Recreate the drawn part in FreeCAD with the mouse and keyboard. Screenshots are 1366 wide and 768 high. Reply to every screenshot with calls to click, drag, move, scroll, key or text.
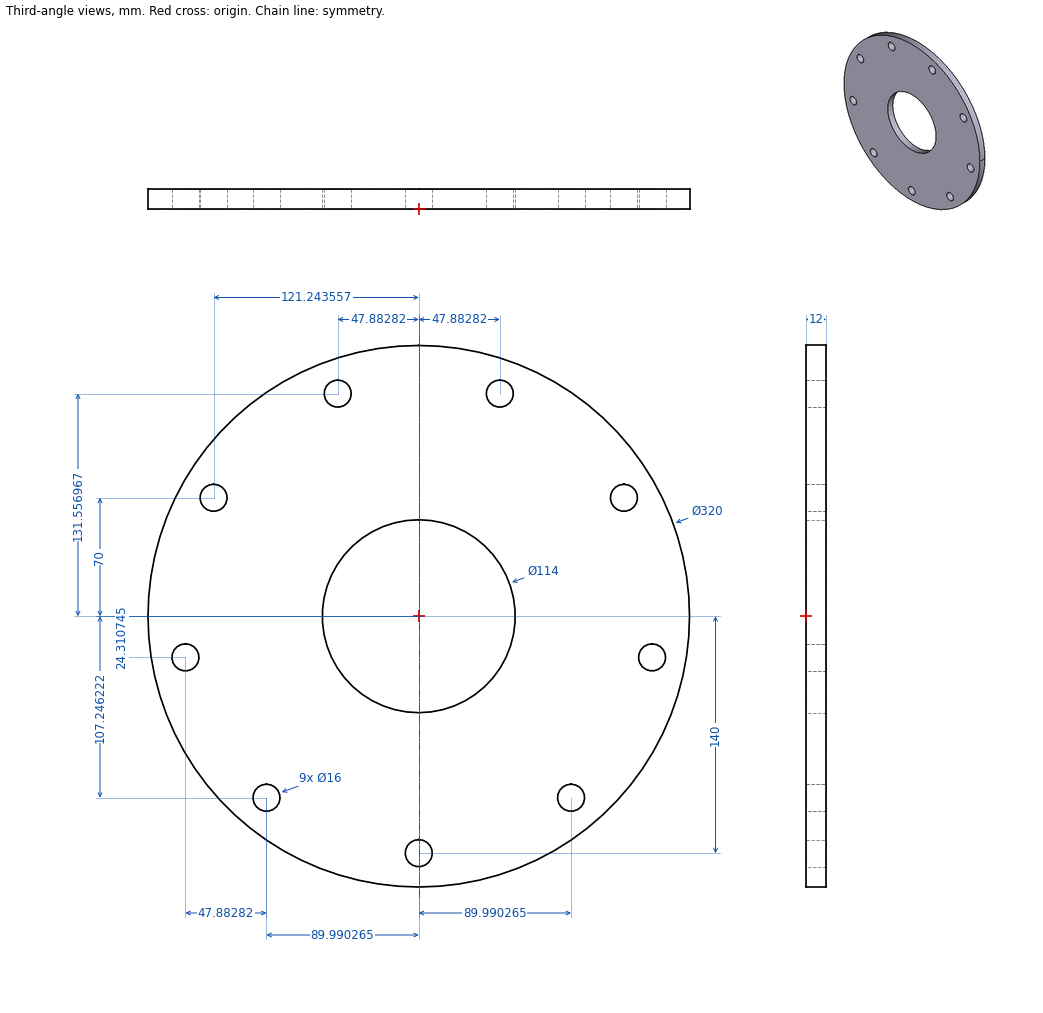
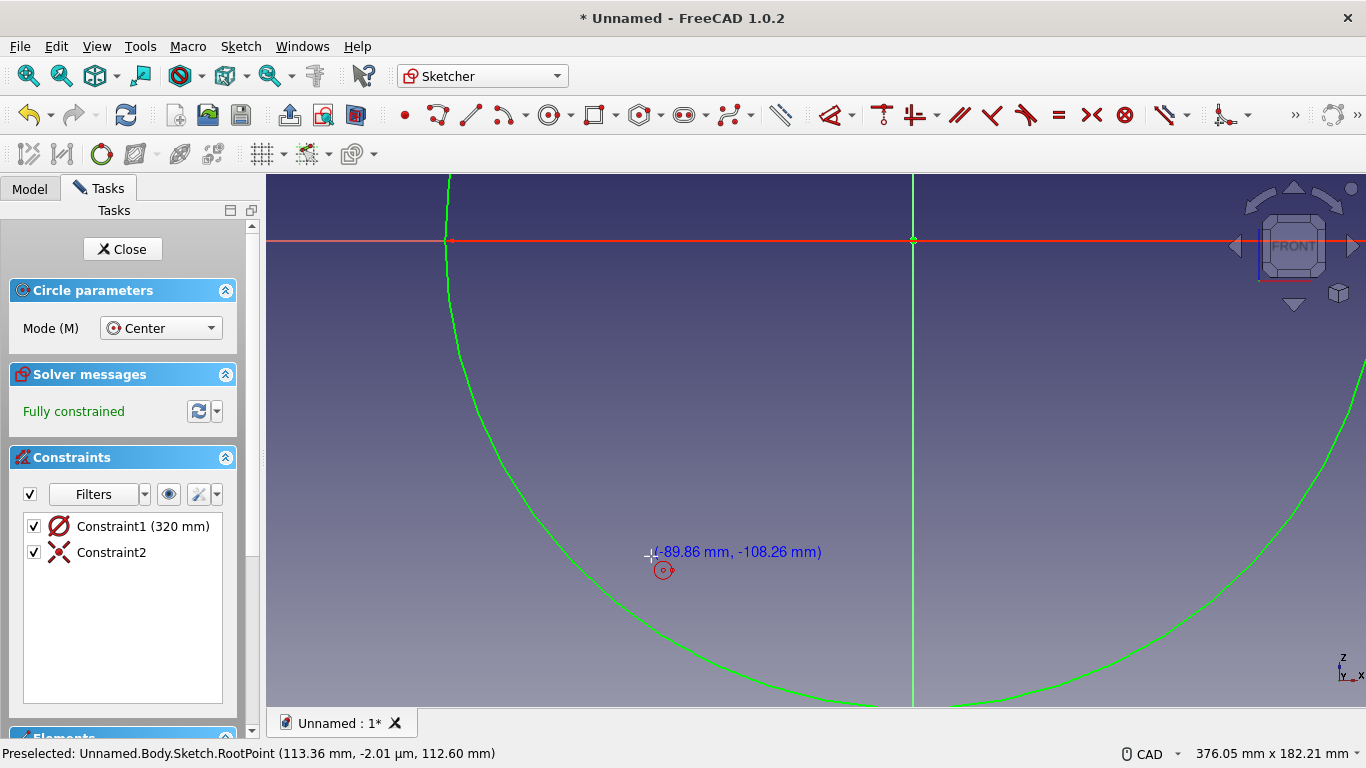
click(650, 555)
move(667, 538)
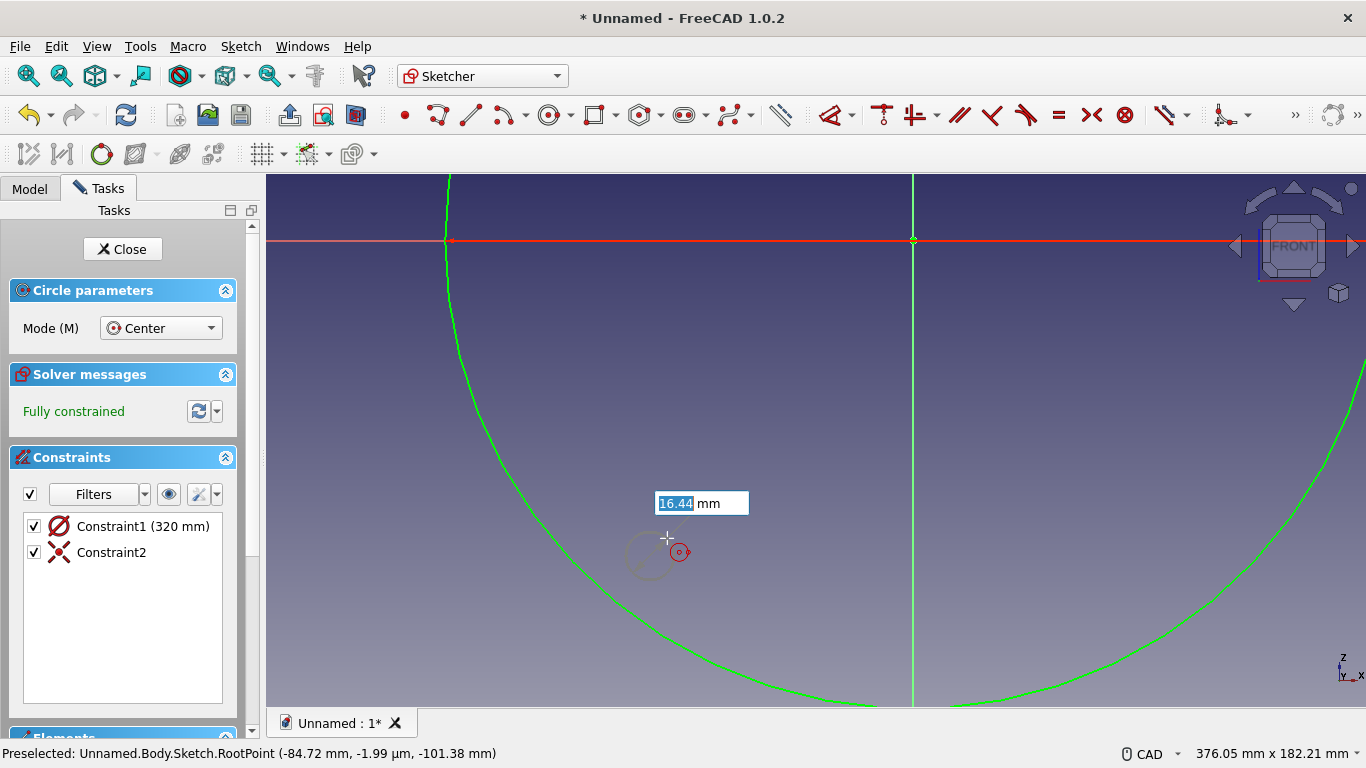
text(16)
key(Return)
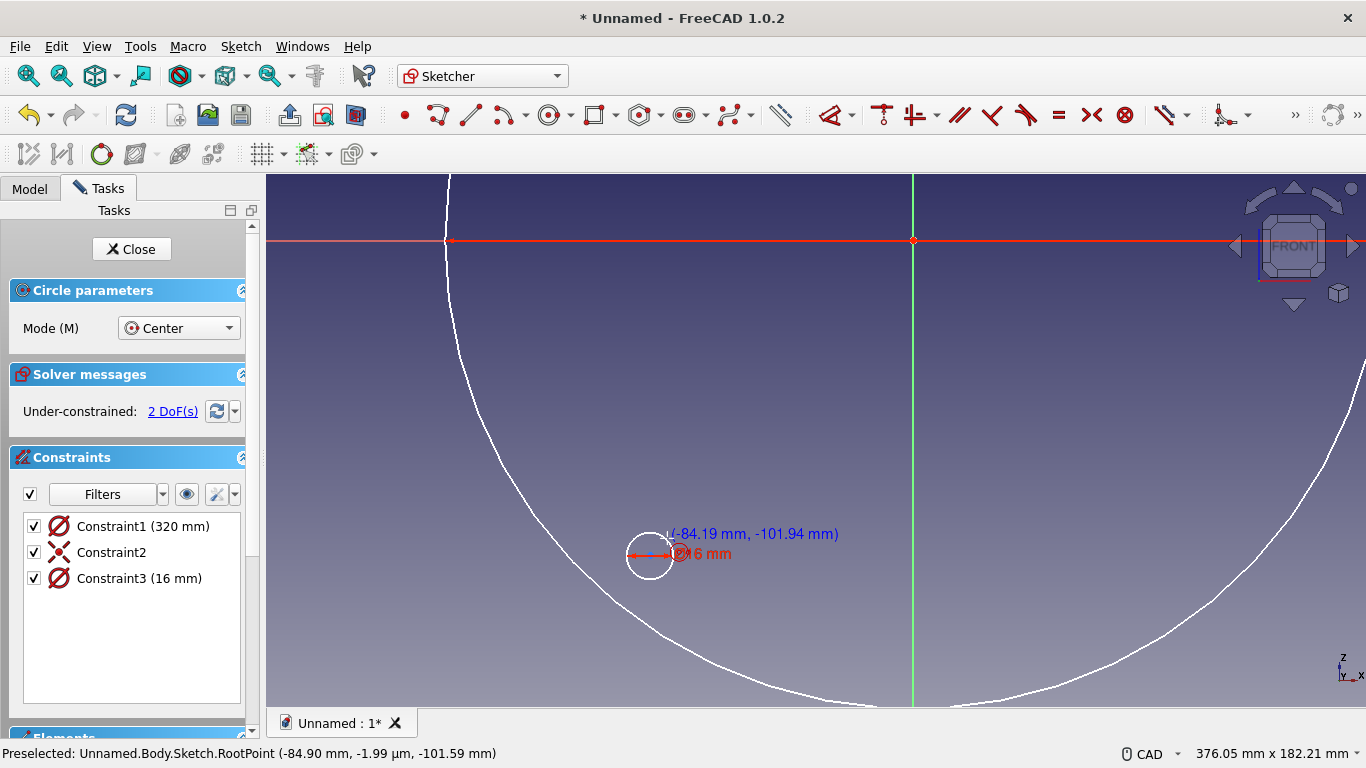
click(510, 312)
move(527, 295)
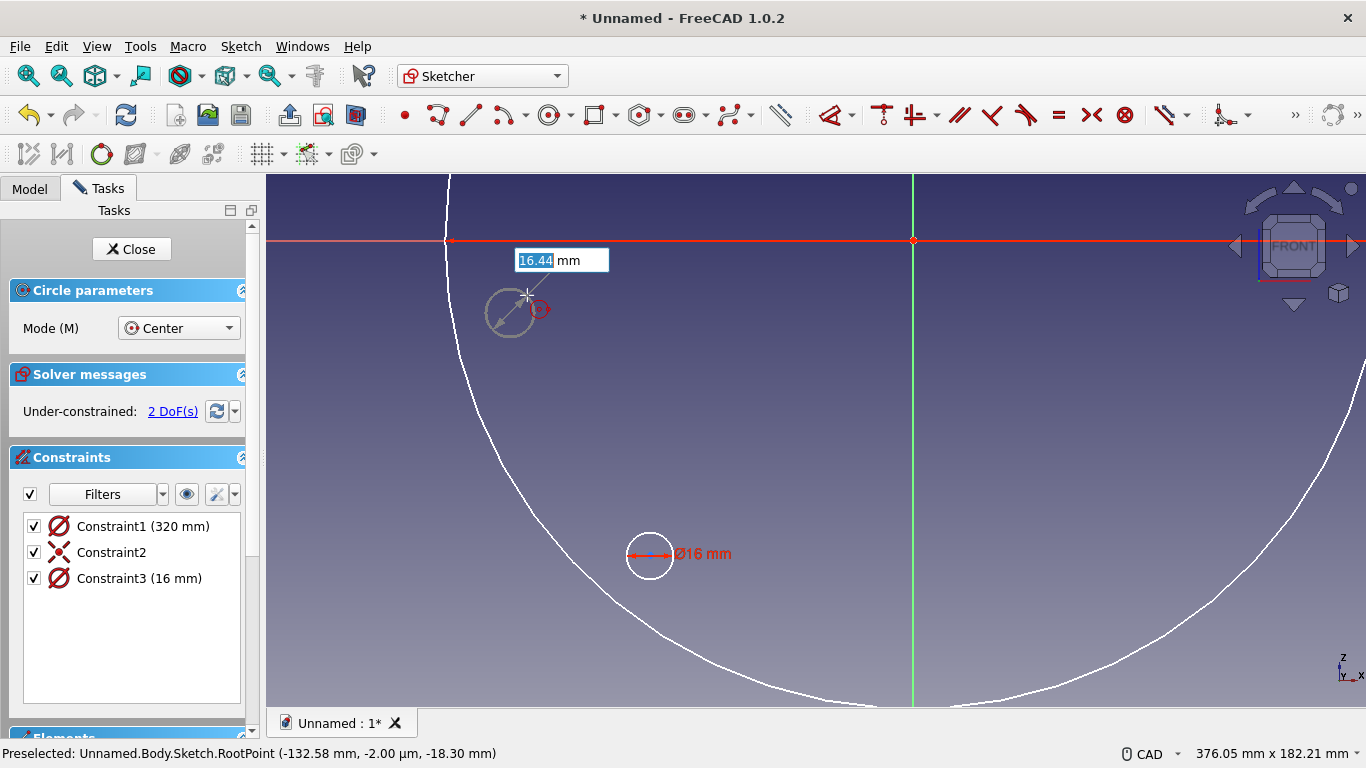
text(16)
key(Return)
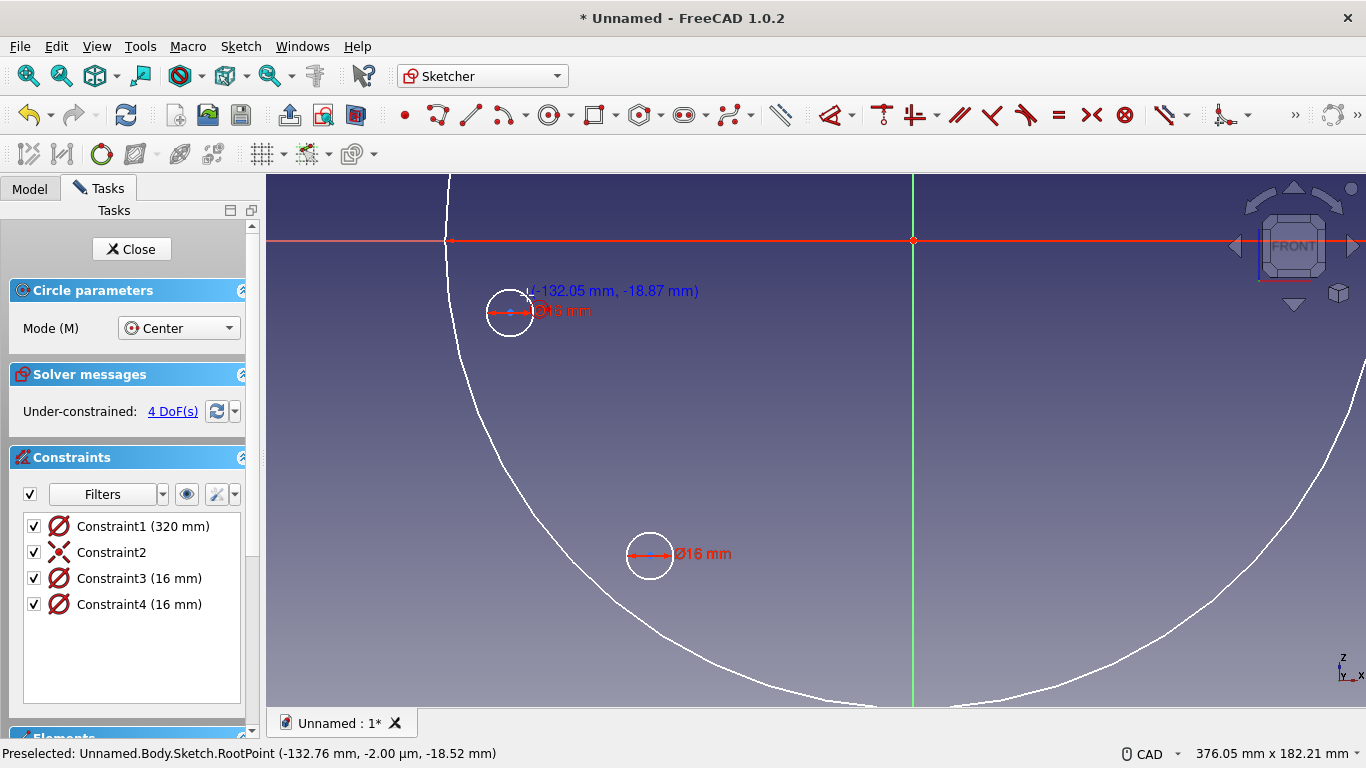
click(913, 650)
move(930, 634)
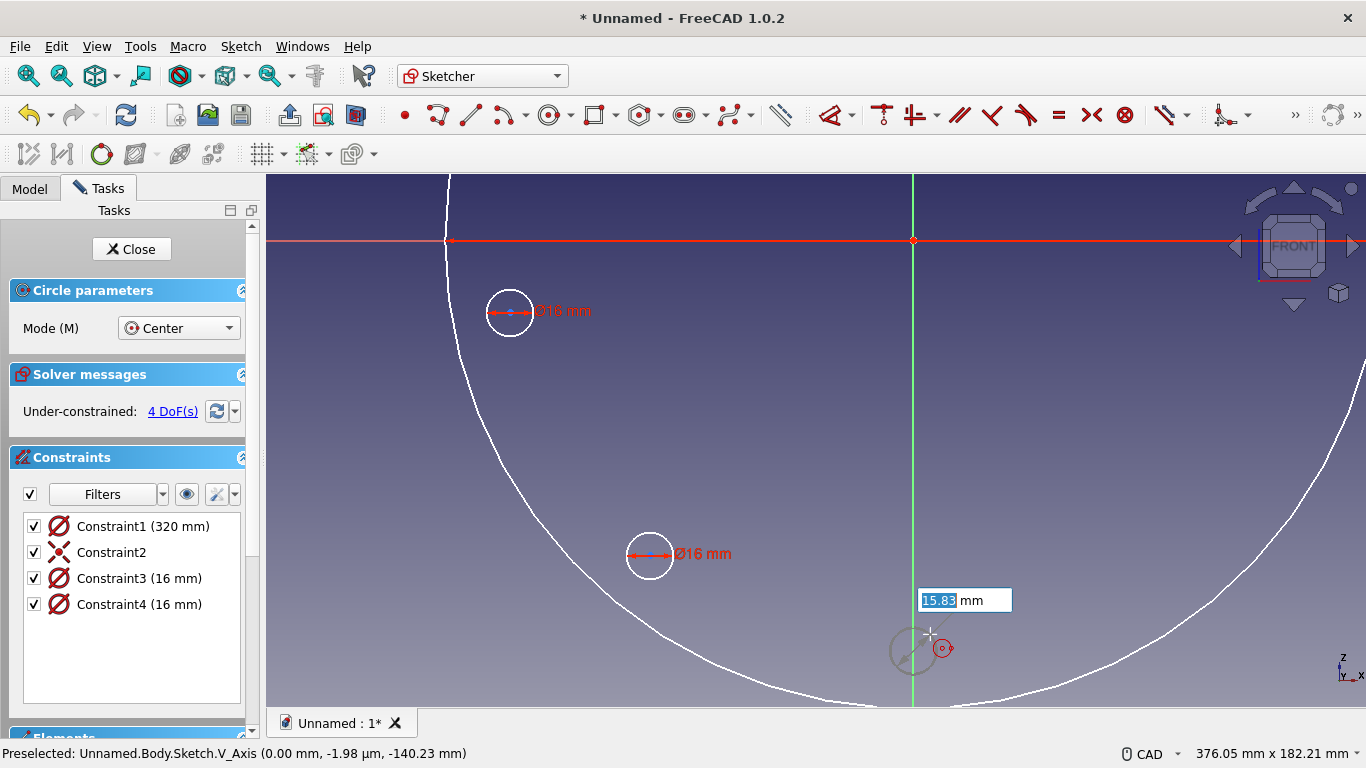
text(16)
key(Return)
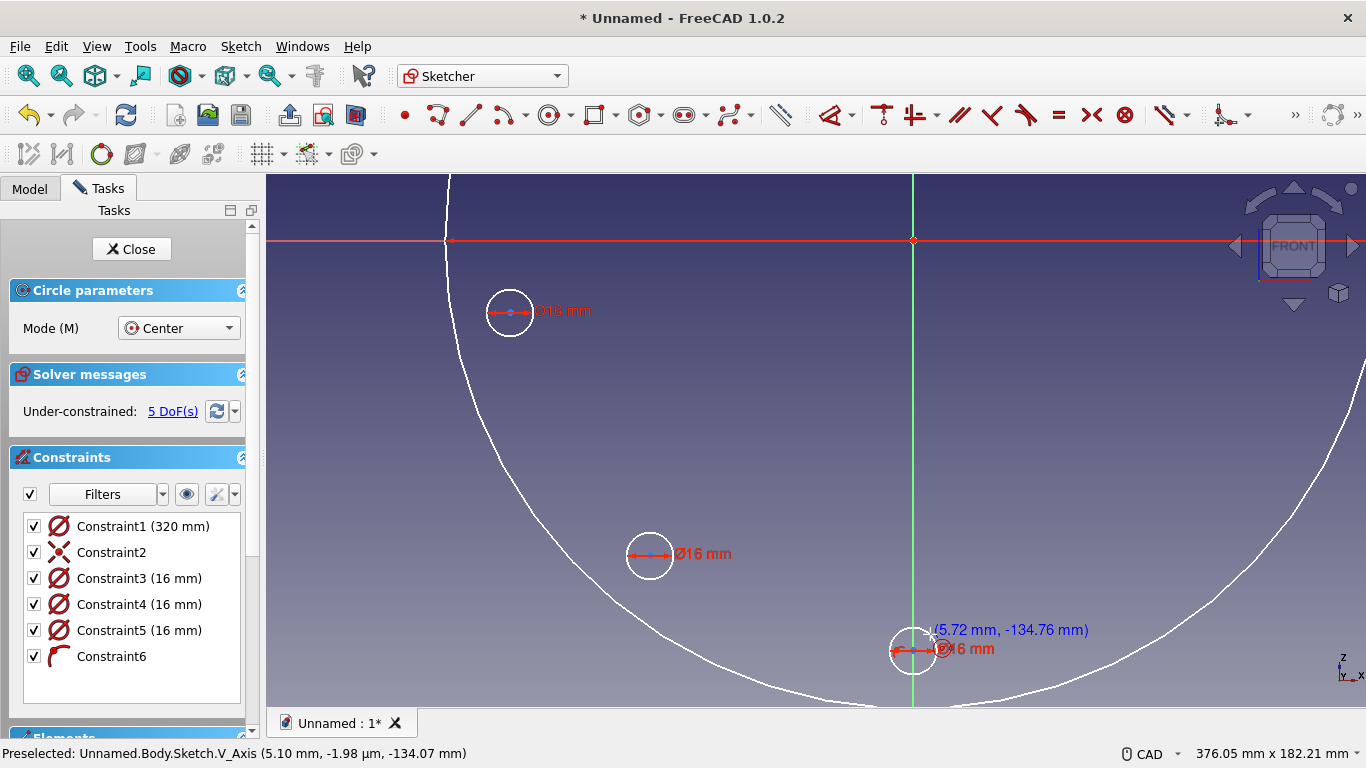
scroll(651, 557, down, 5)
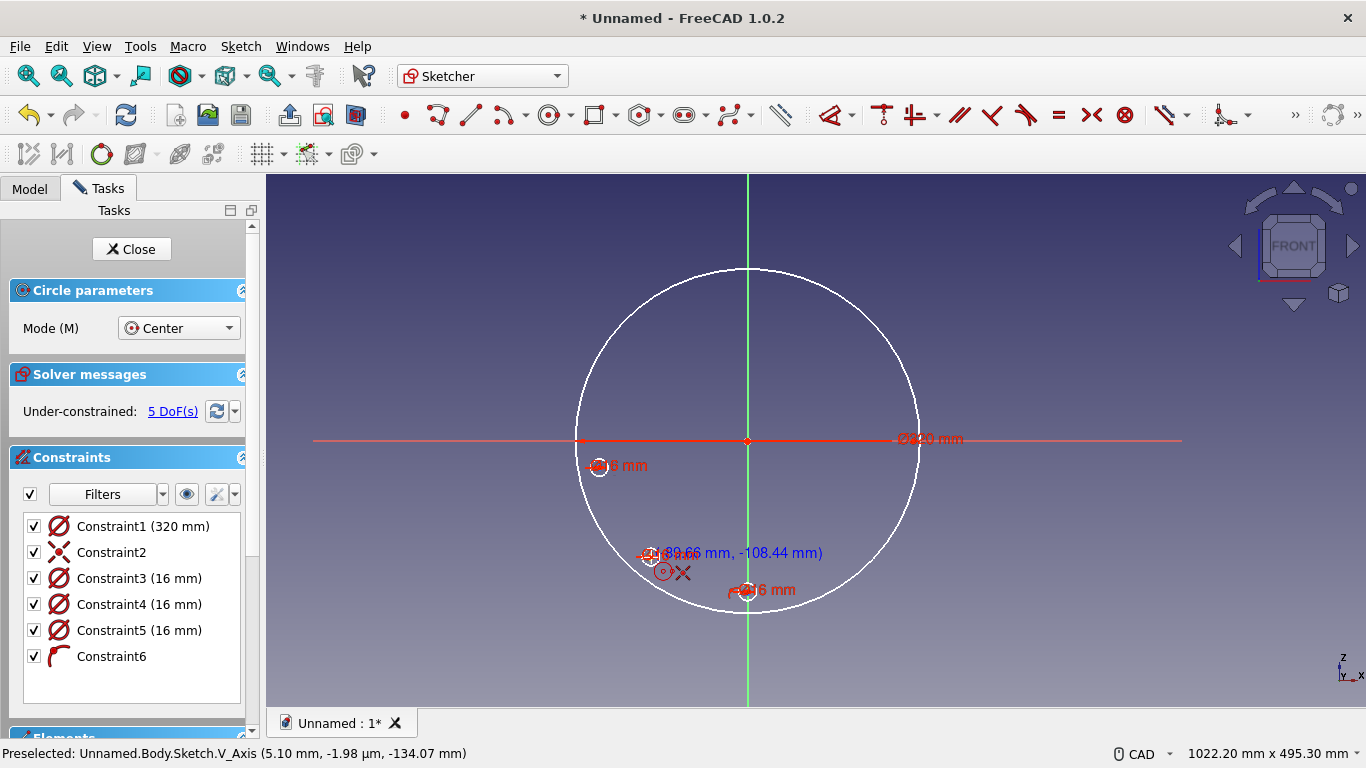
scroll(617, 366, up, 5)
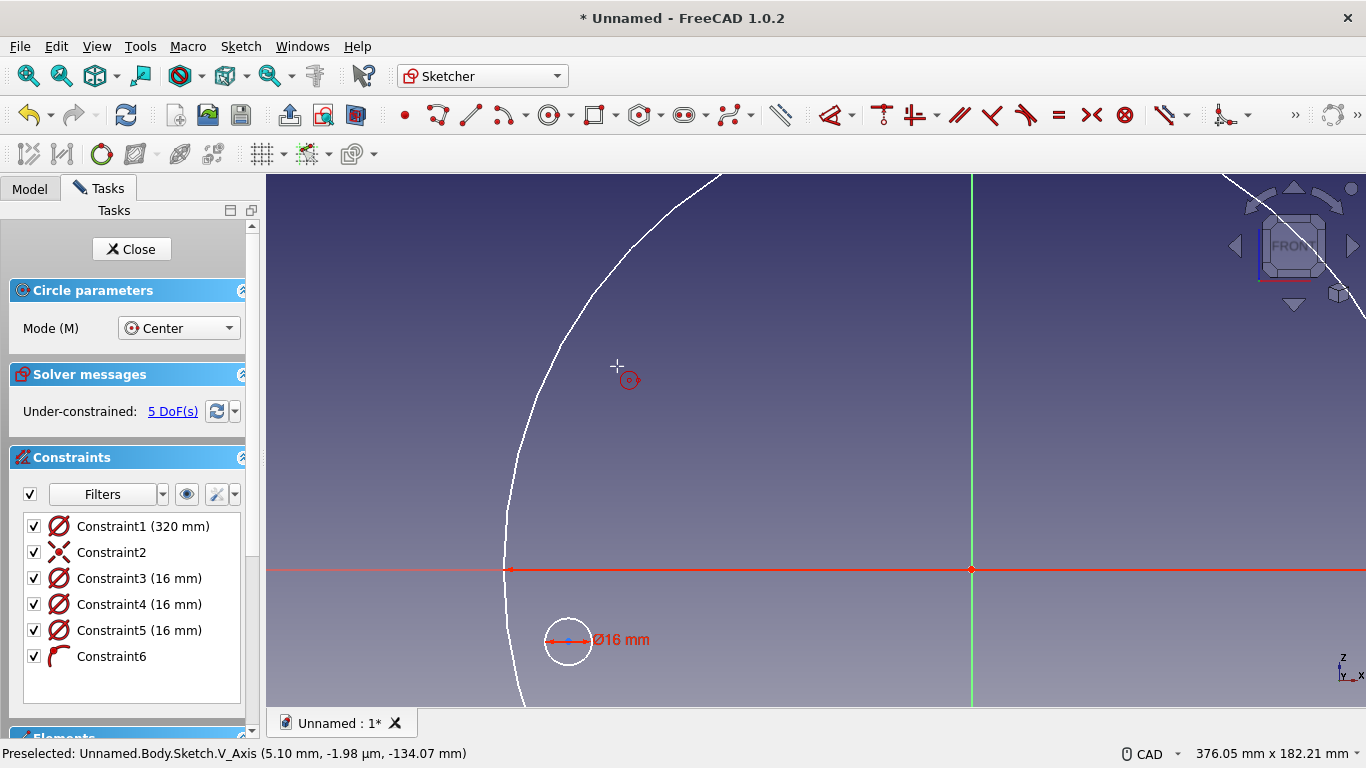
click(617, 365)
move(634, 348)